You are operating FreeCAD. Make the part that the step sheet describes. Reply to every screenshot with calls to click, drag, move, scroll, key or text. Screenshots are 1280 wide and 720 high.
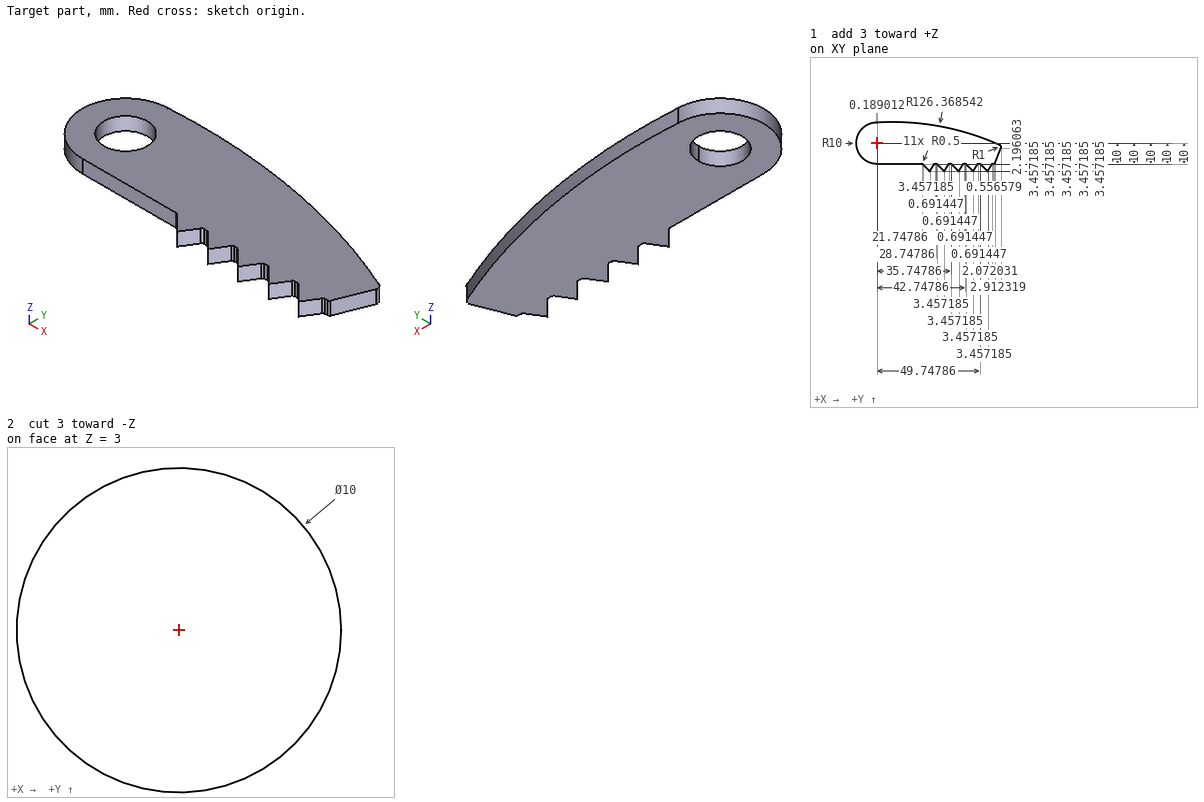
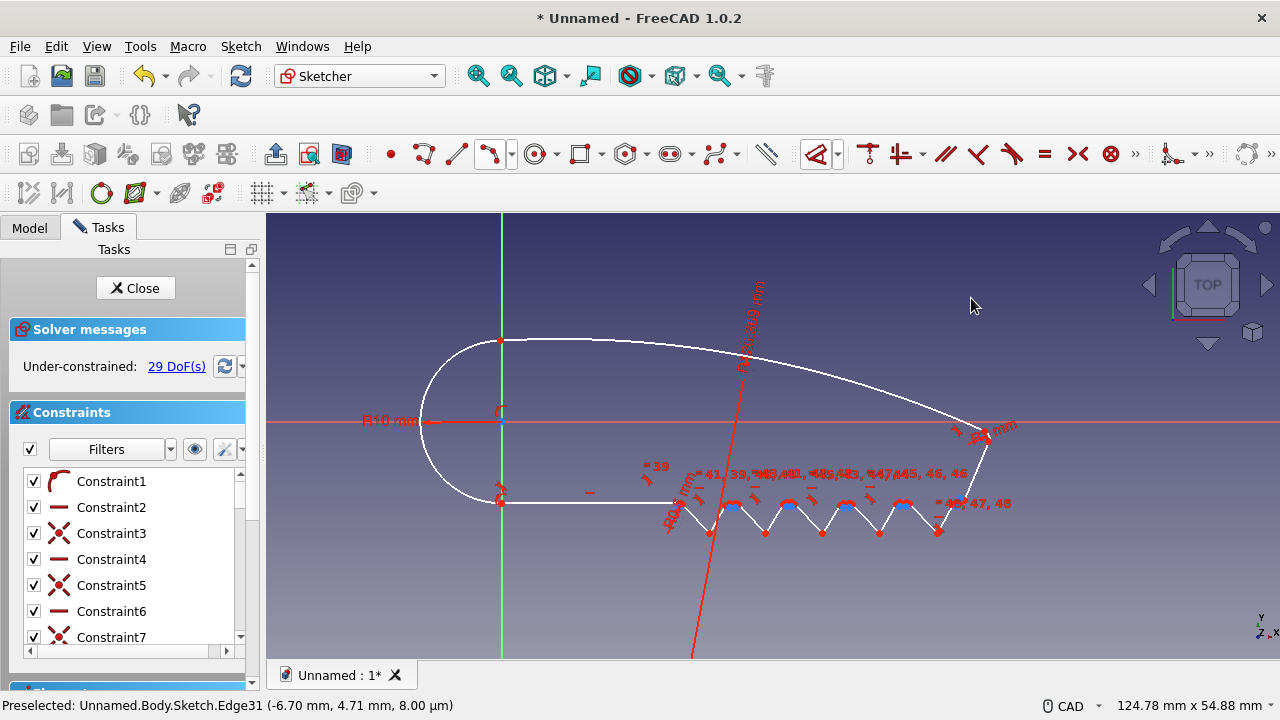
scroll(729, 503, up, 6)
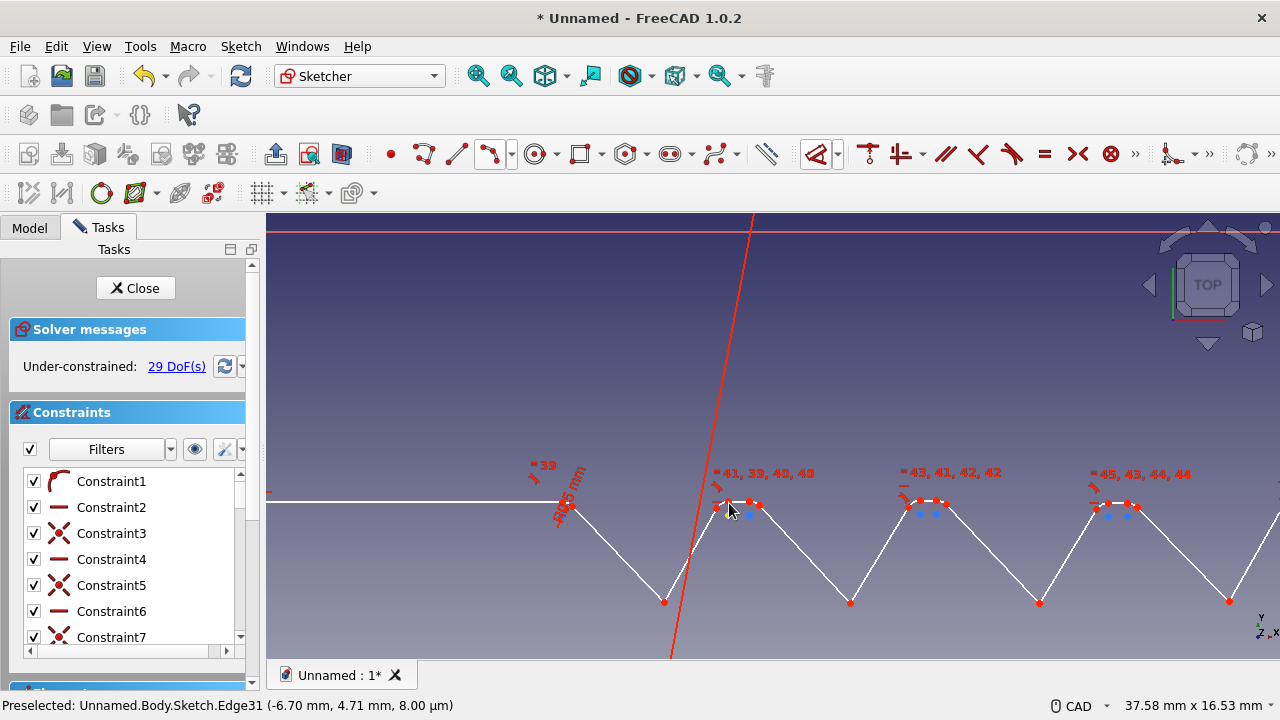
click(729, 502)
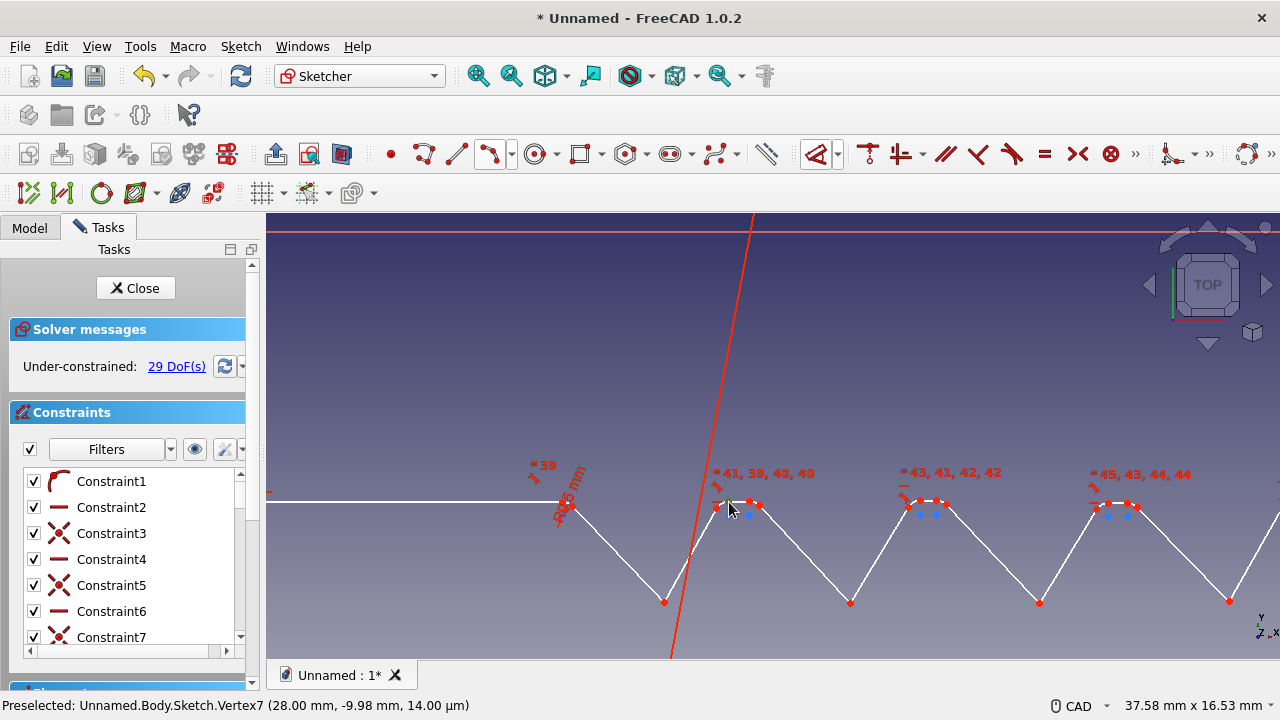
key(i)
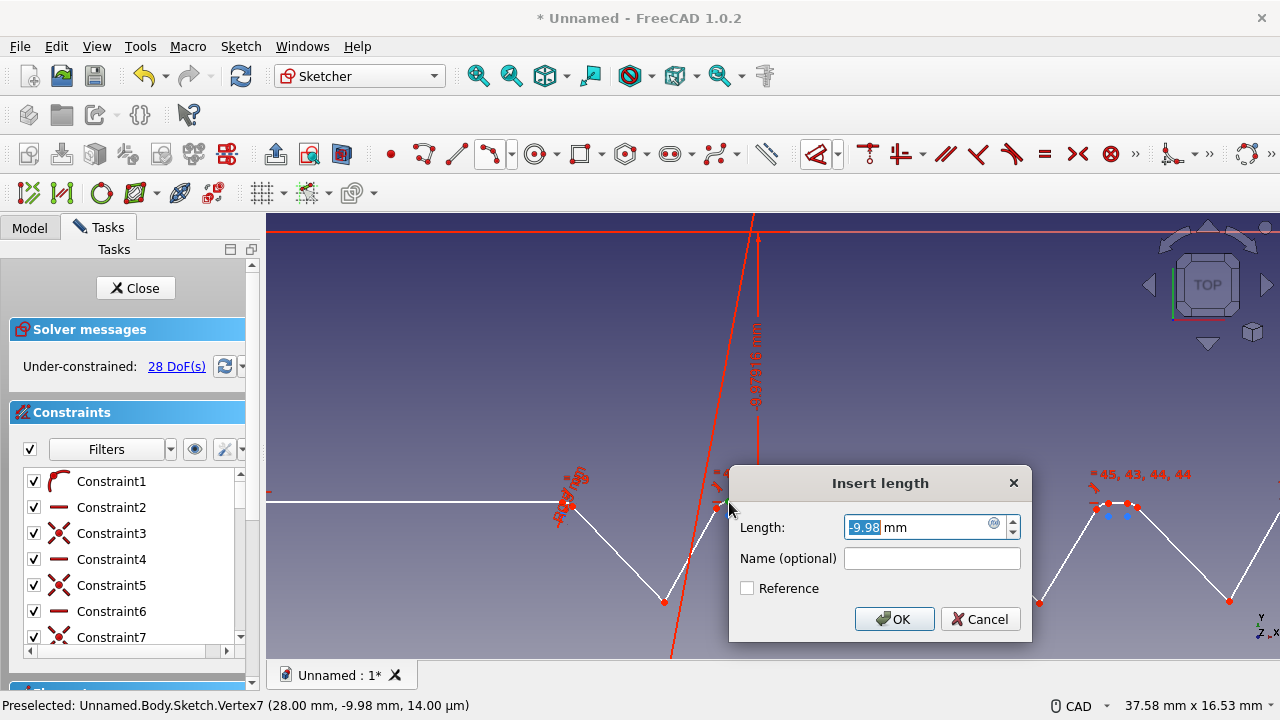
text(-10)
key(Return)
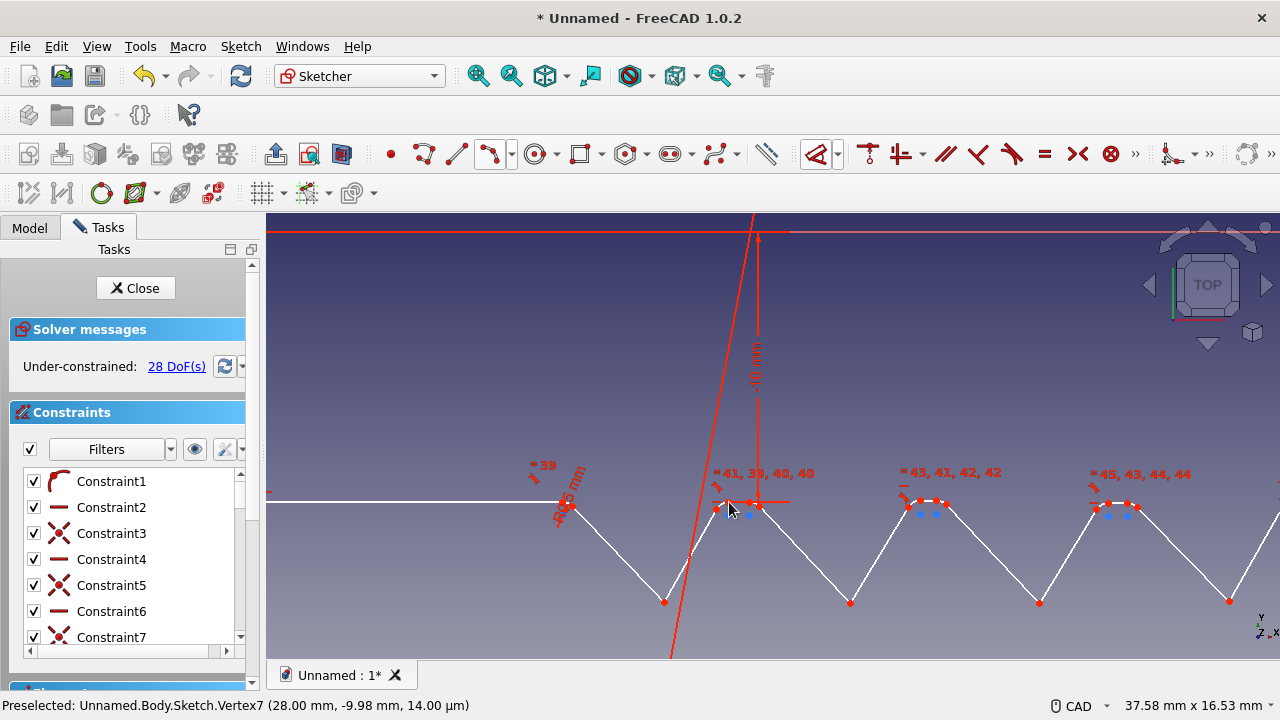
click(920, 501)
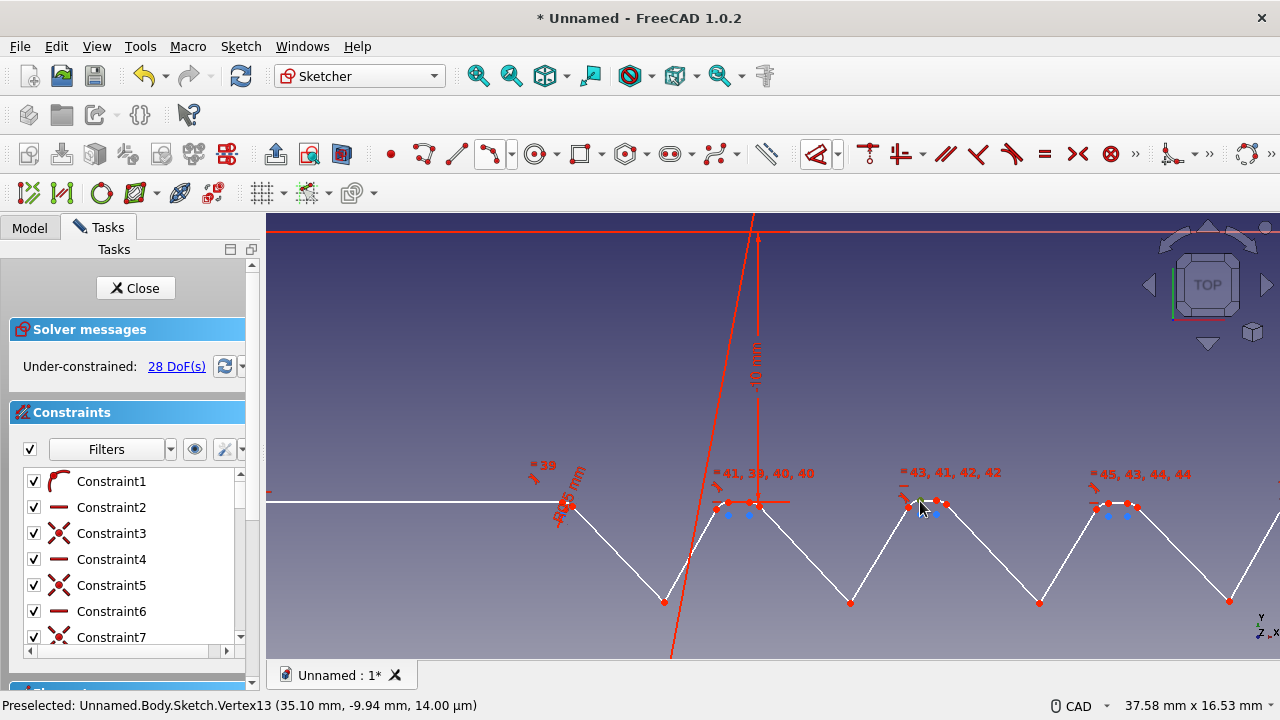
click(838, 154)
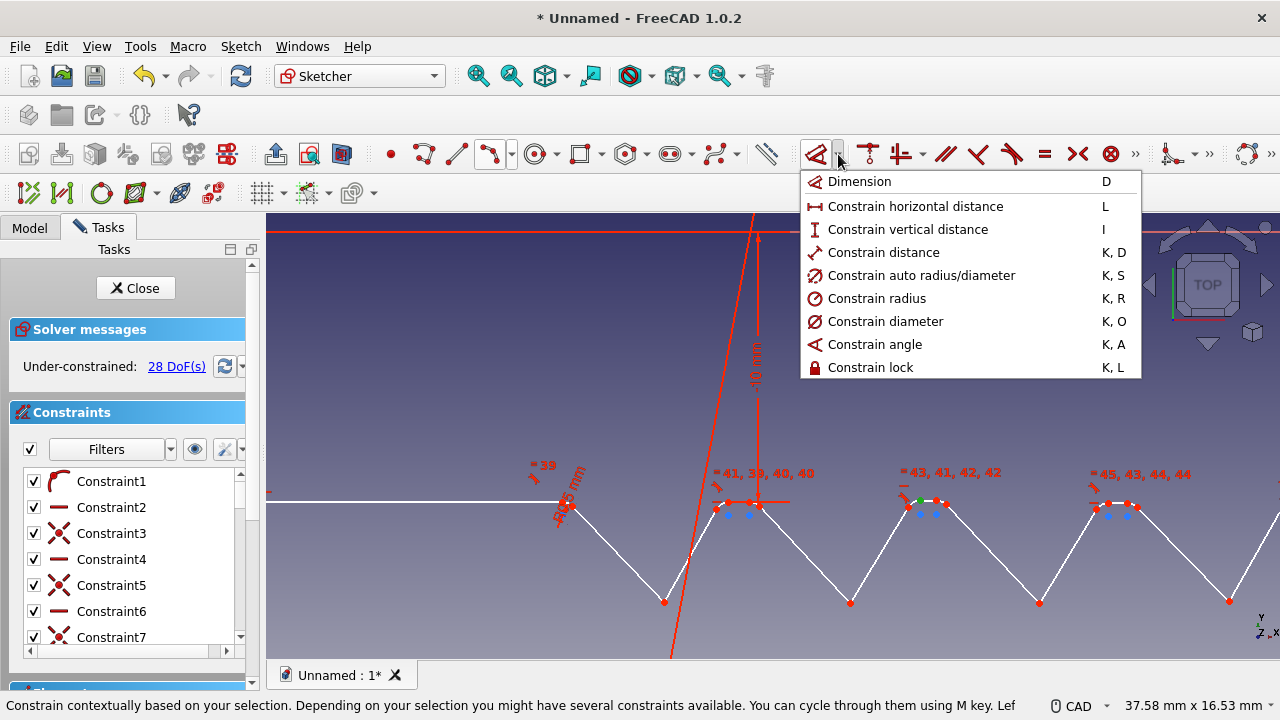
click(971, 230)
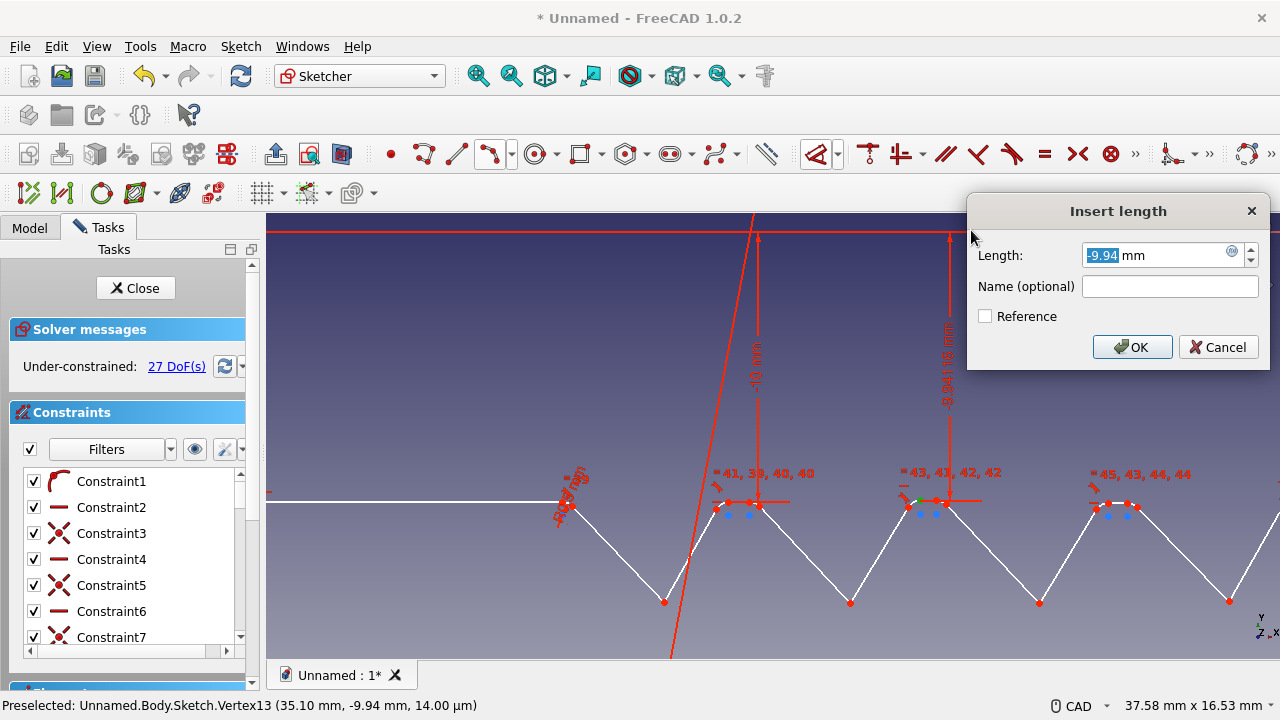
text(-10)
key(Return)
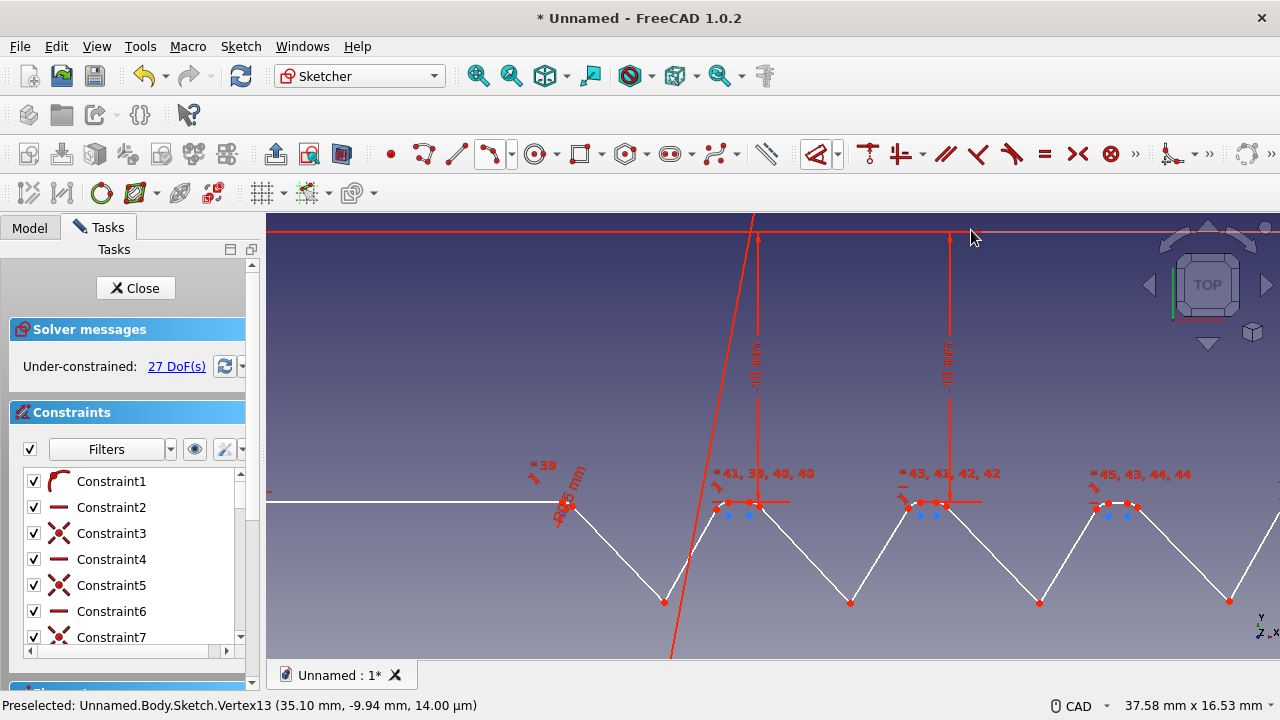
click(1108, 503)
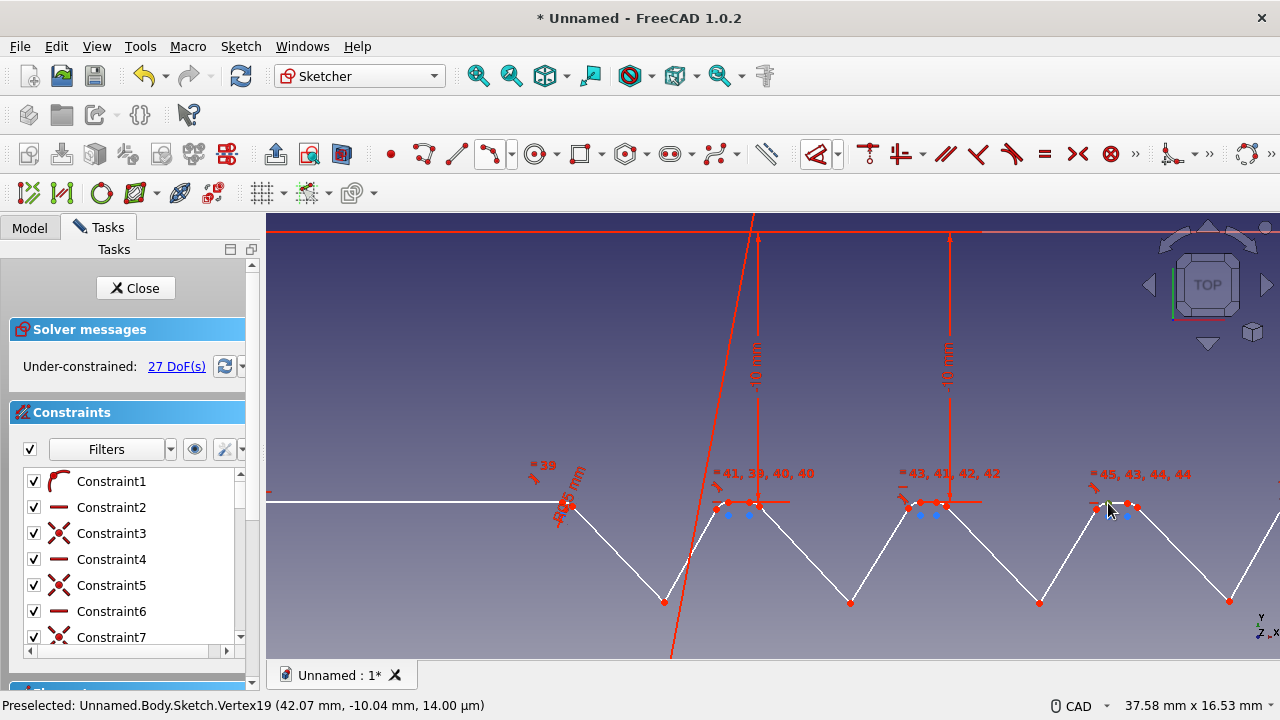
key(i)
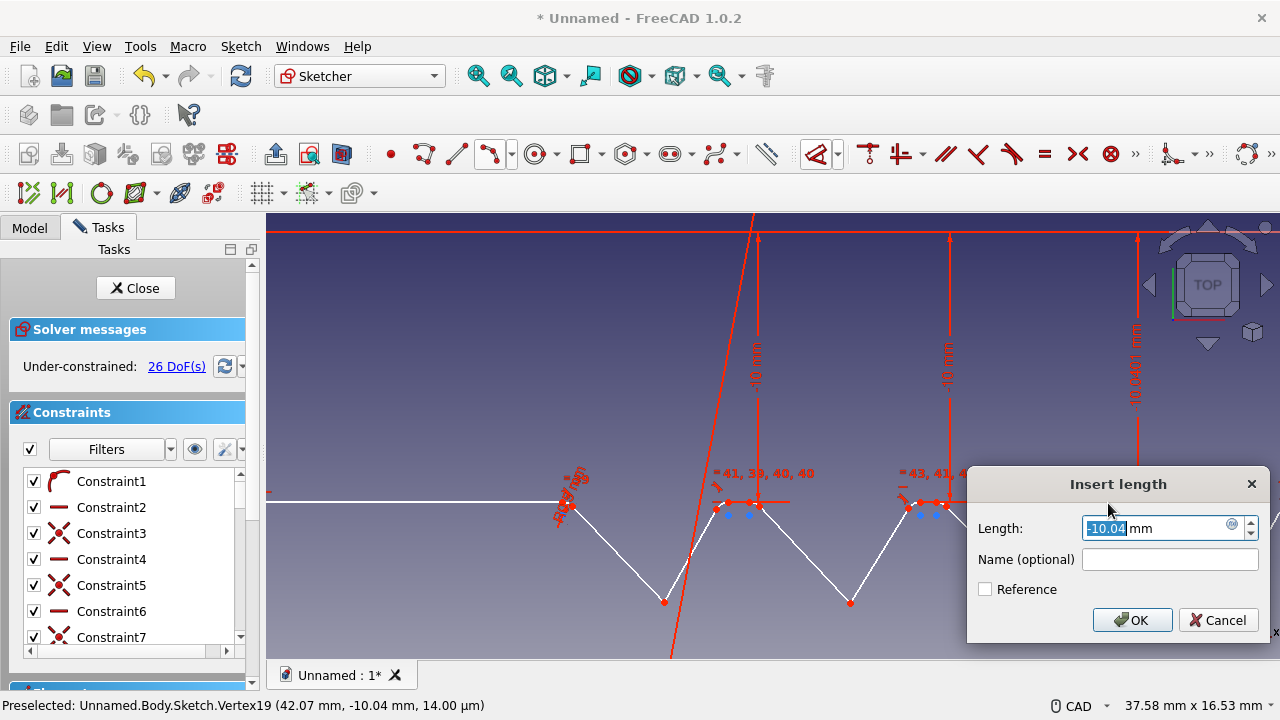
text(-10)
key(Return)